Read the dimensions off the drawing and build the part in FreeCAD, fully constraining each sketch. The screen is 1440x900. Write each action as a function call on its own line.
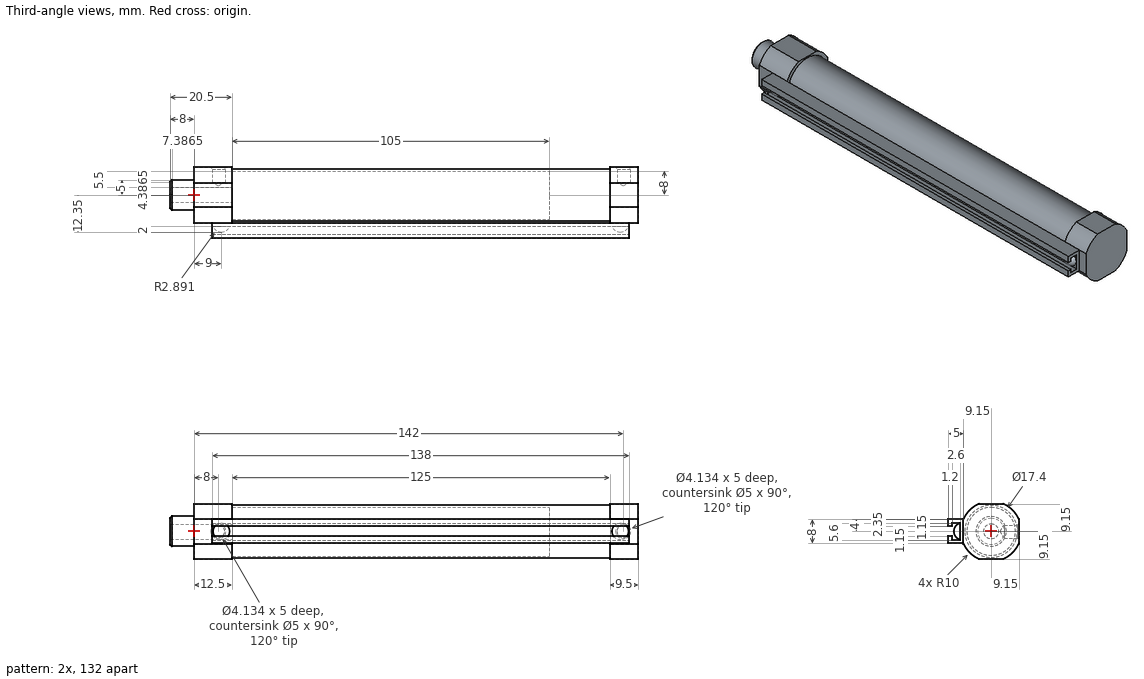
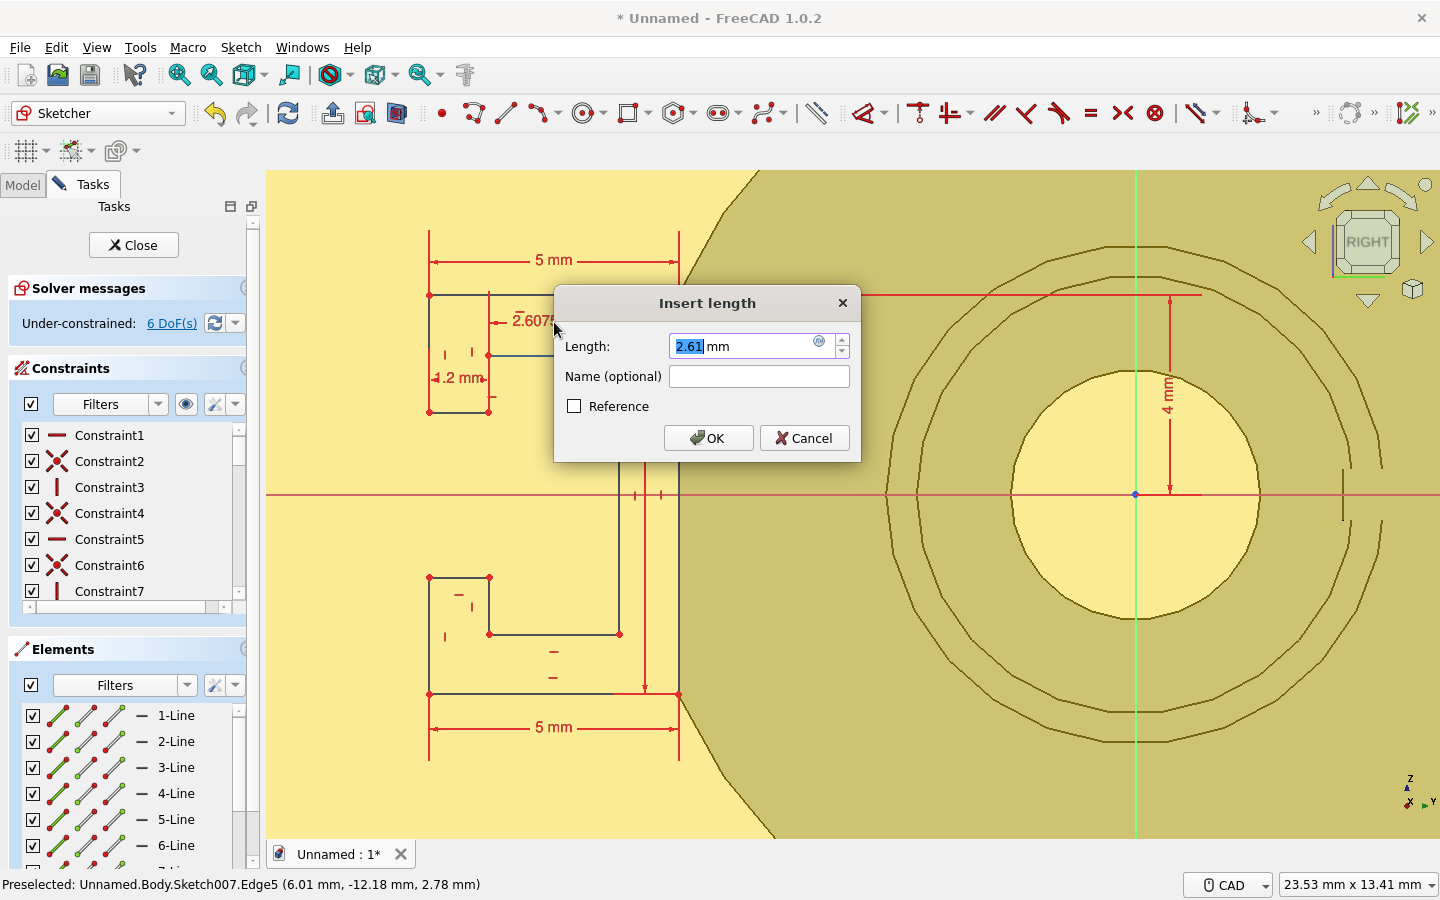
text(2.6)
key(Return)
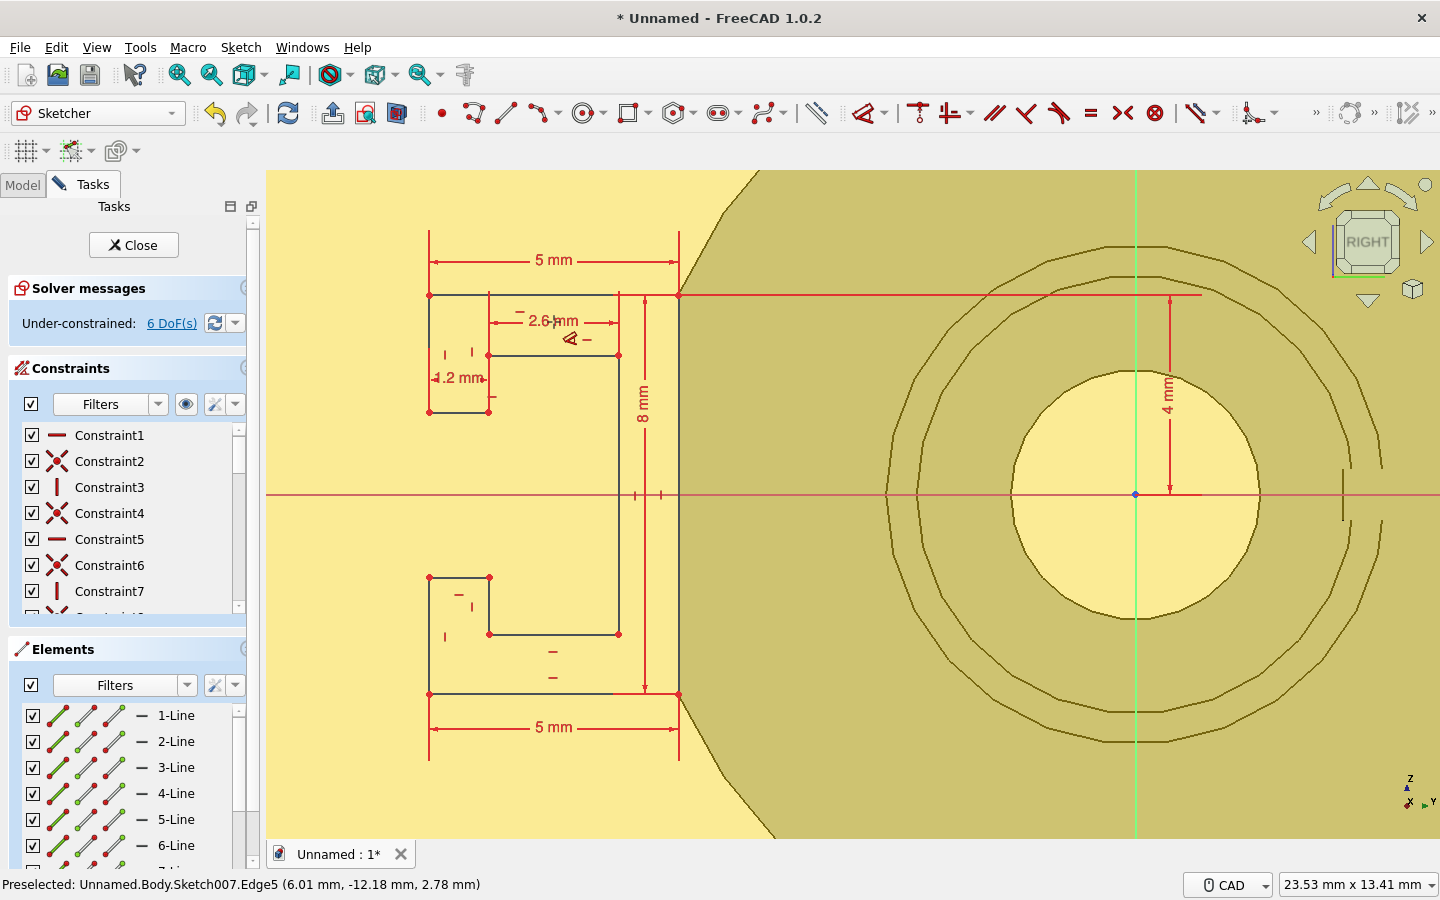
click(619, 440)
click(585, 431)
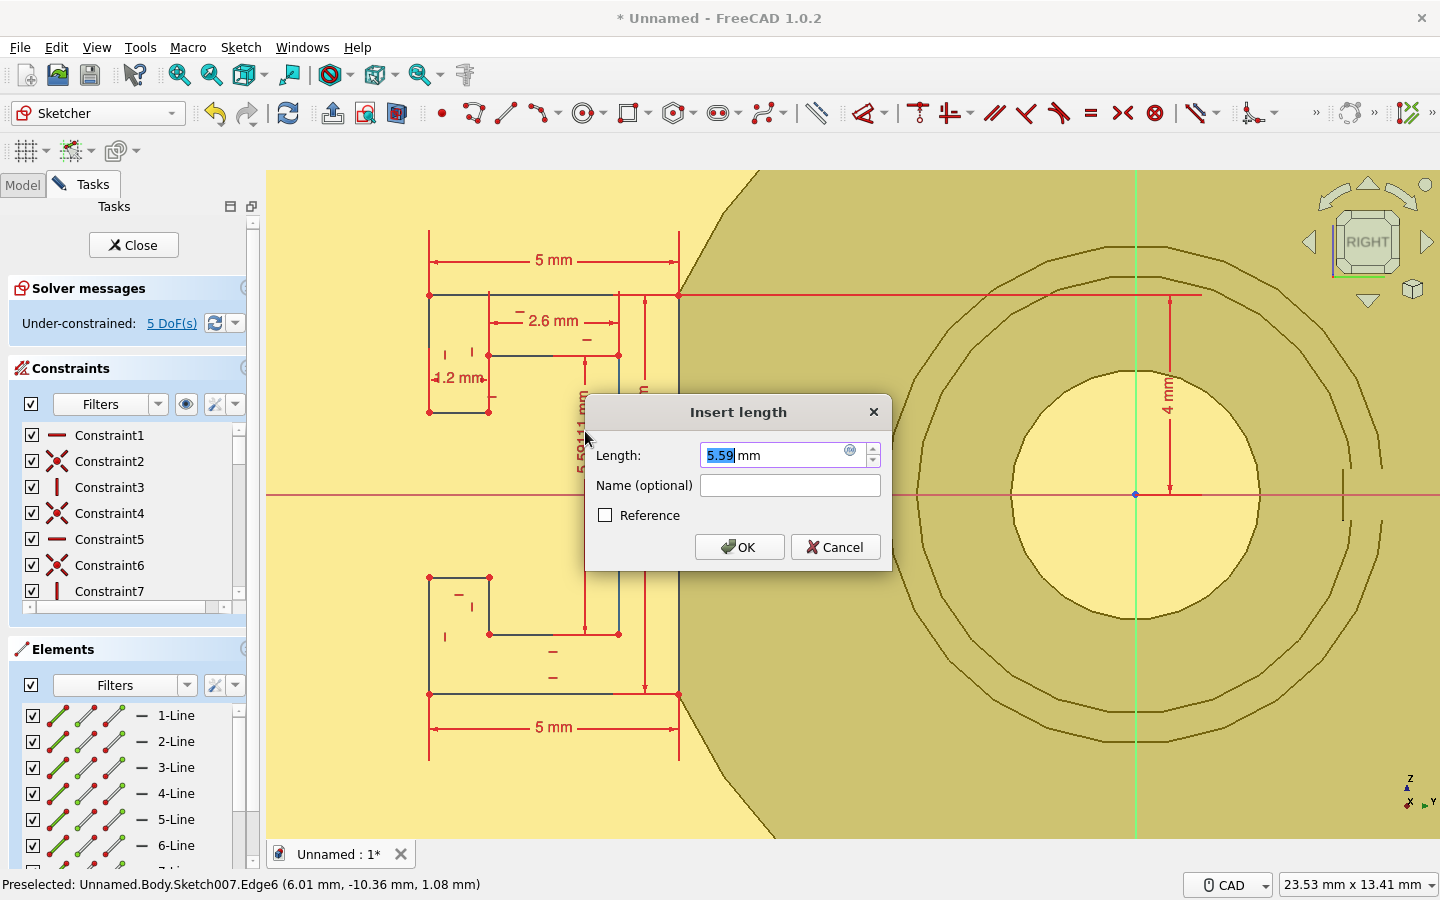
text(5.6)
key(Return)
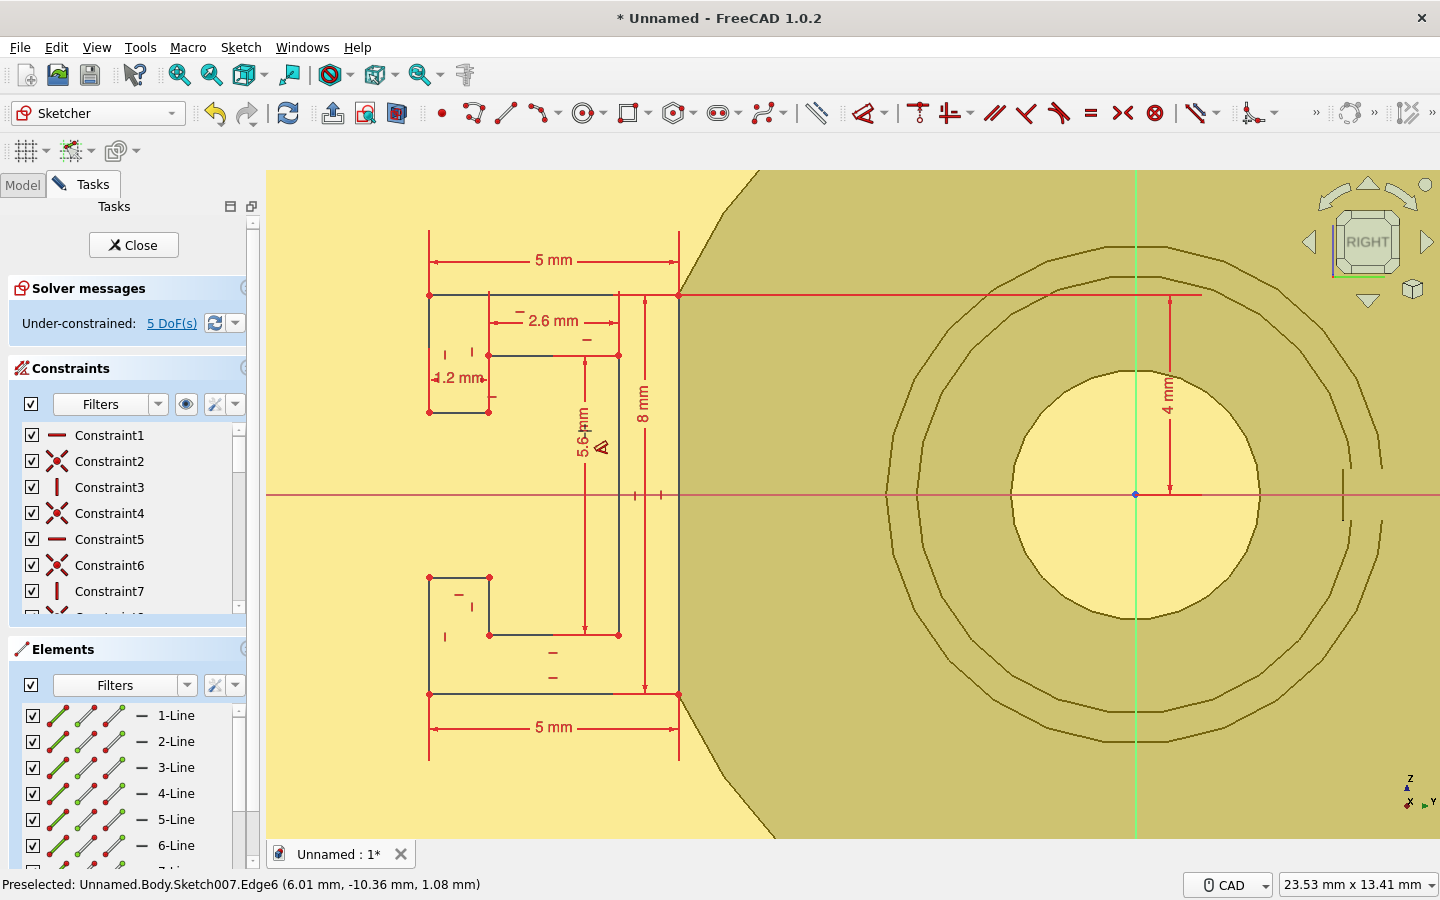
click(580, 635)
click(554, 669)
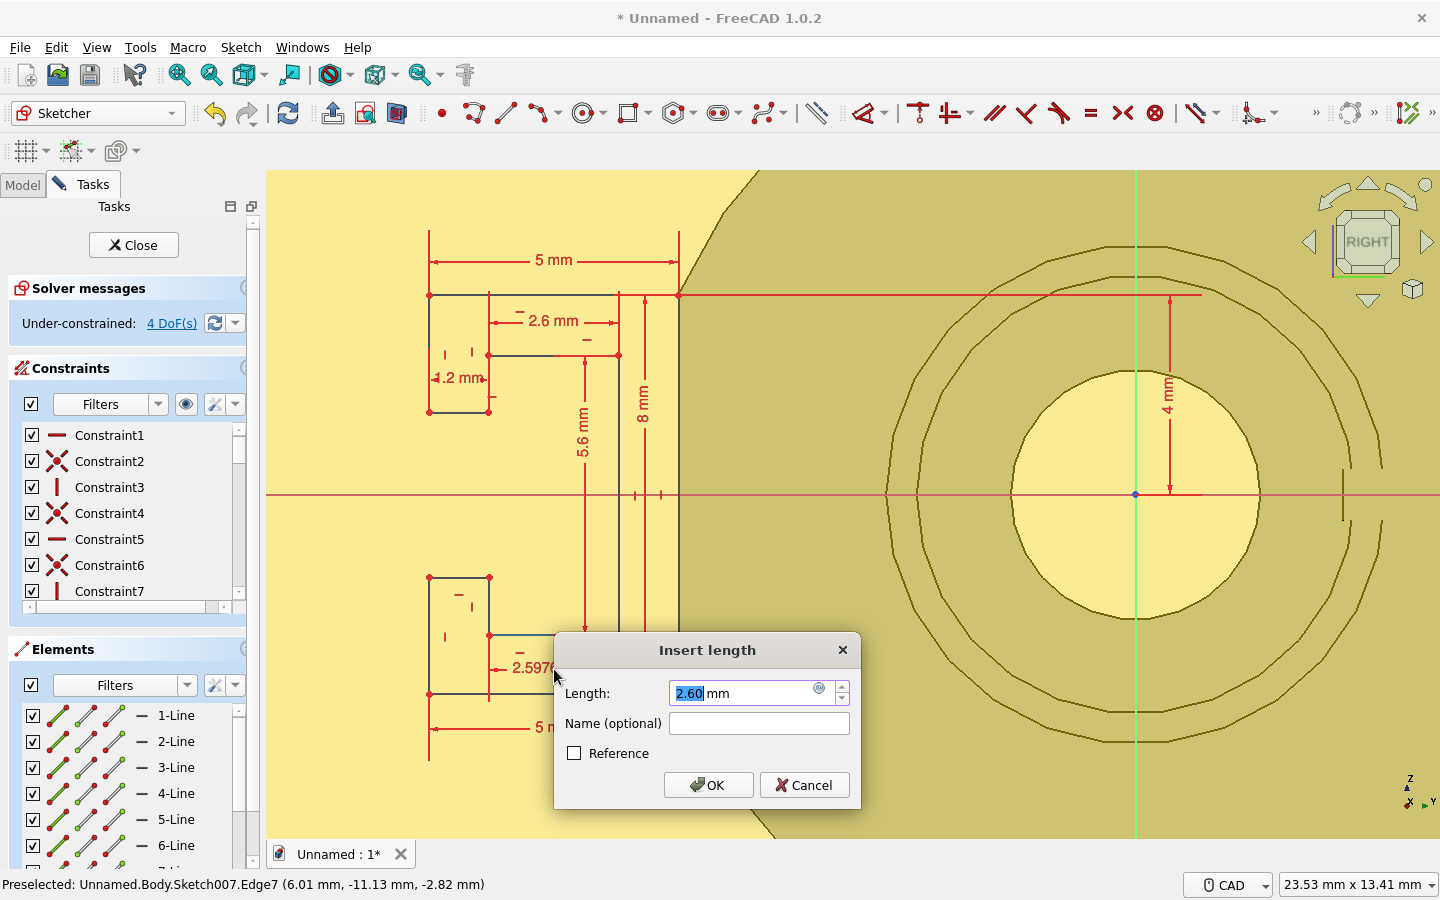
text(2.6)
key(Return)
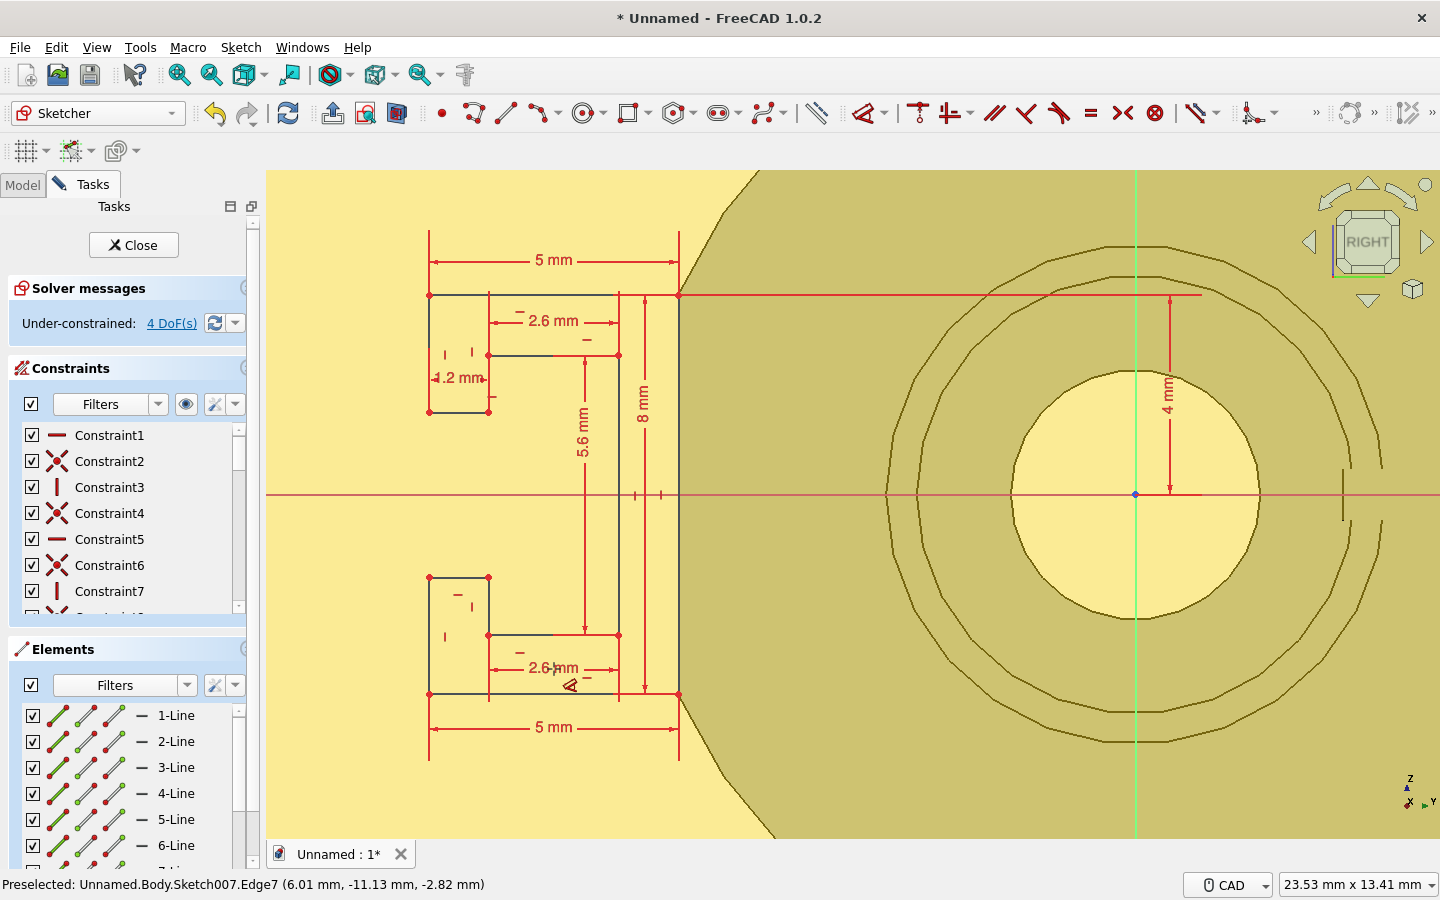
click(429, 330)
click(395, 354)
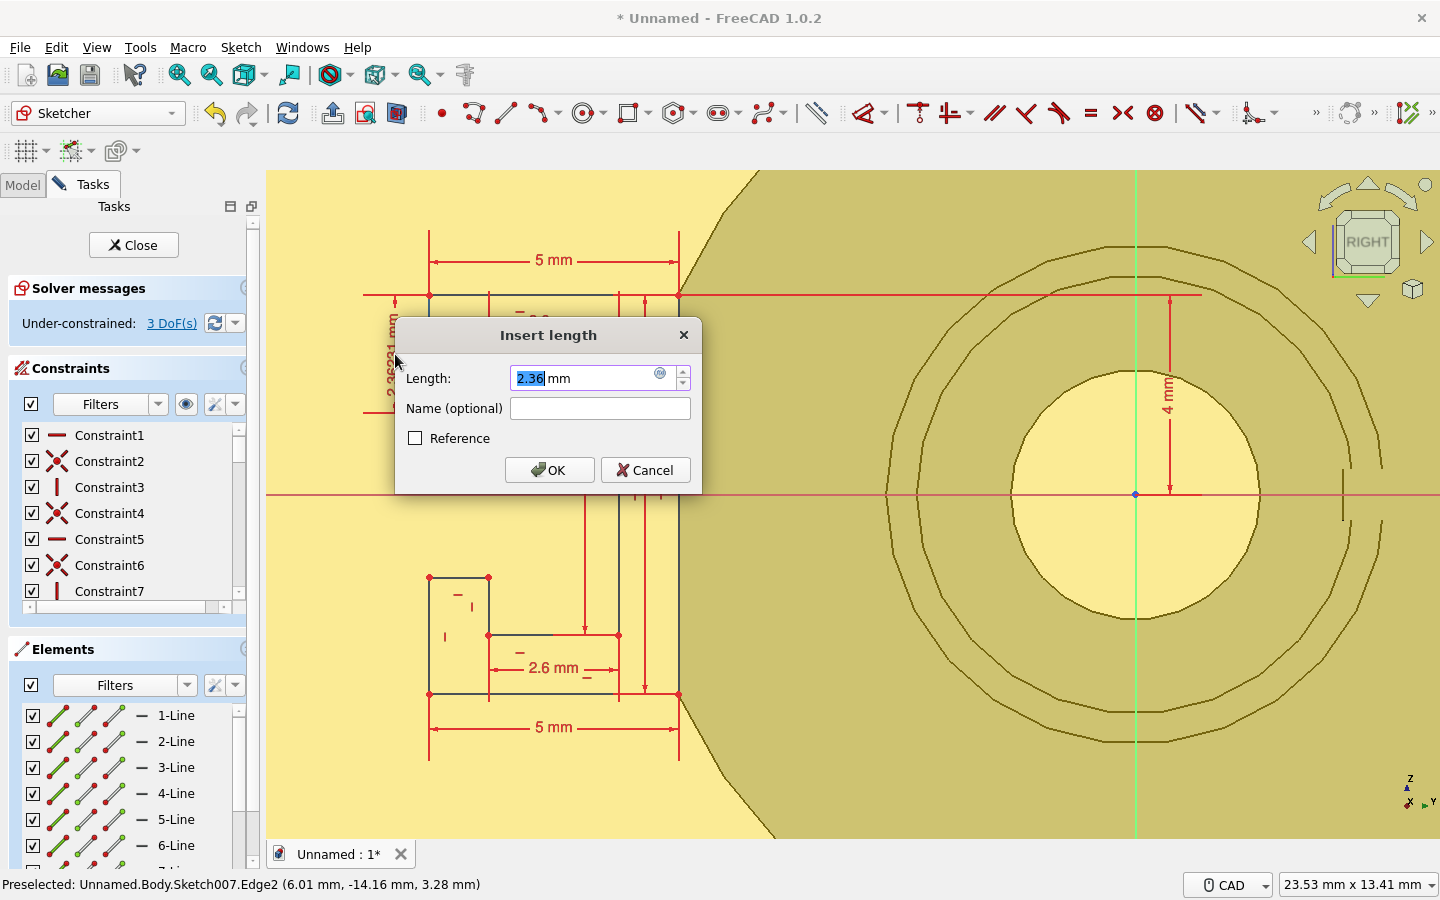
text(2.35)
key(Return)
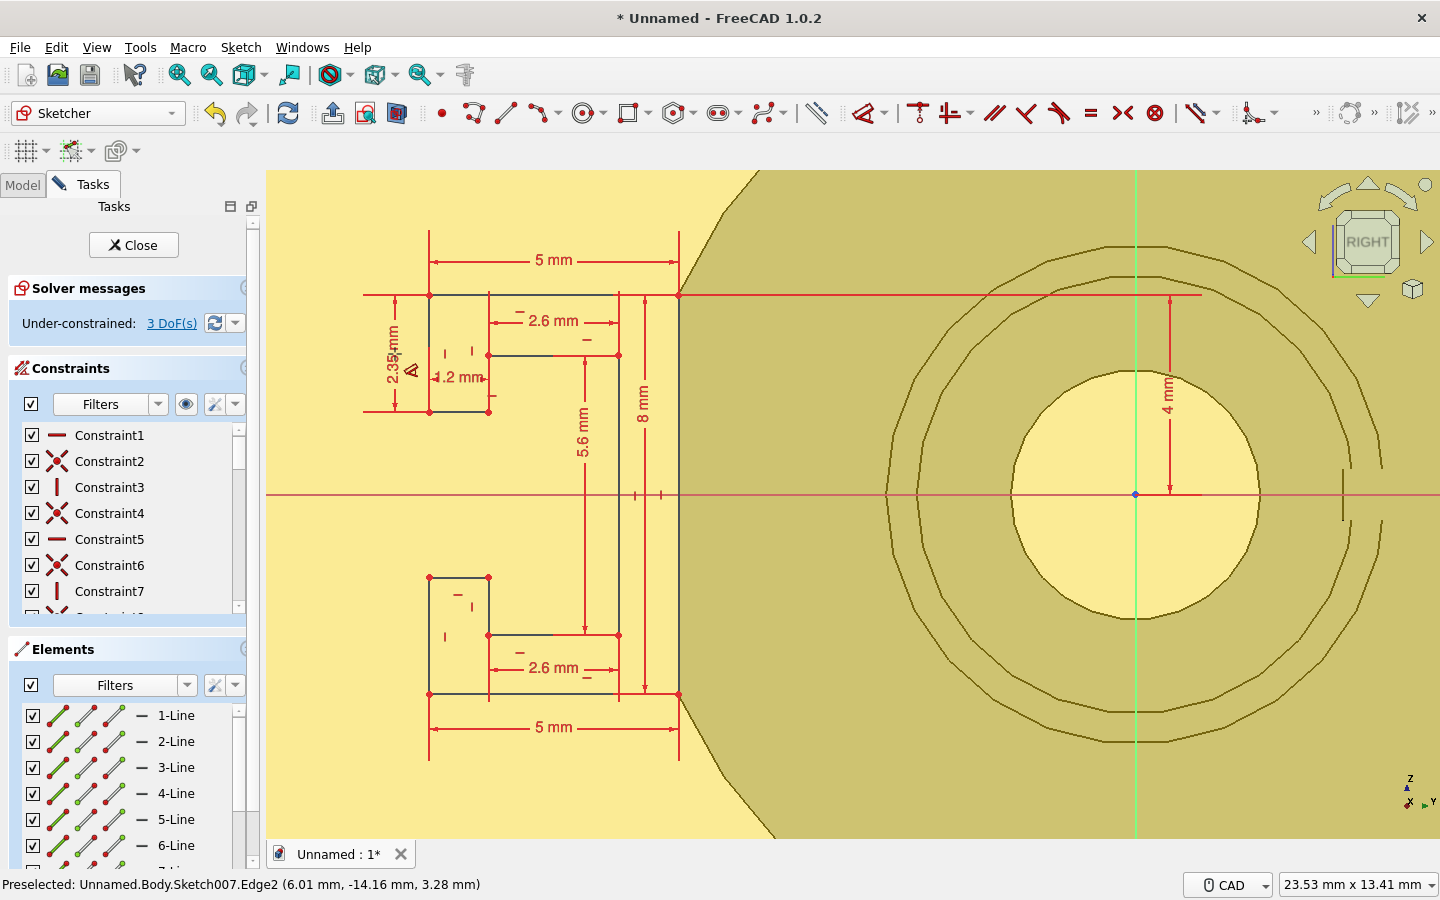
click(489, 395)
click(523, 404)